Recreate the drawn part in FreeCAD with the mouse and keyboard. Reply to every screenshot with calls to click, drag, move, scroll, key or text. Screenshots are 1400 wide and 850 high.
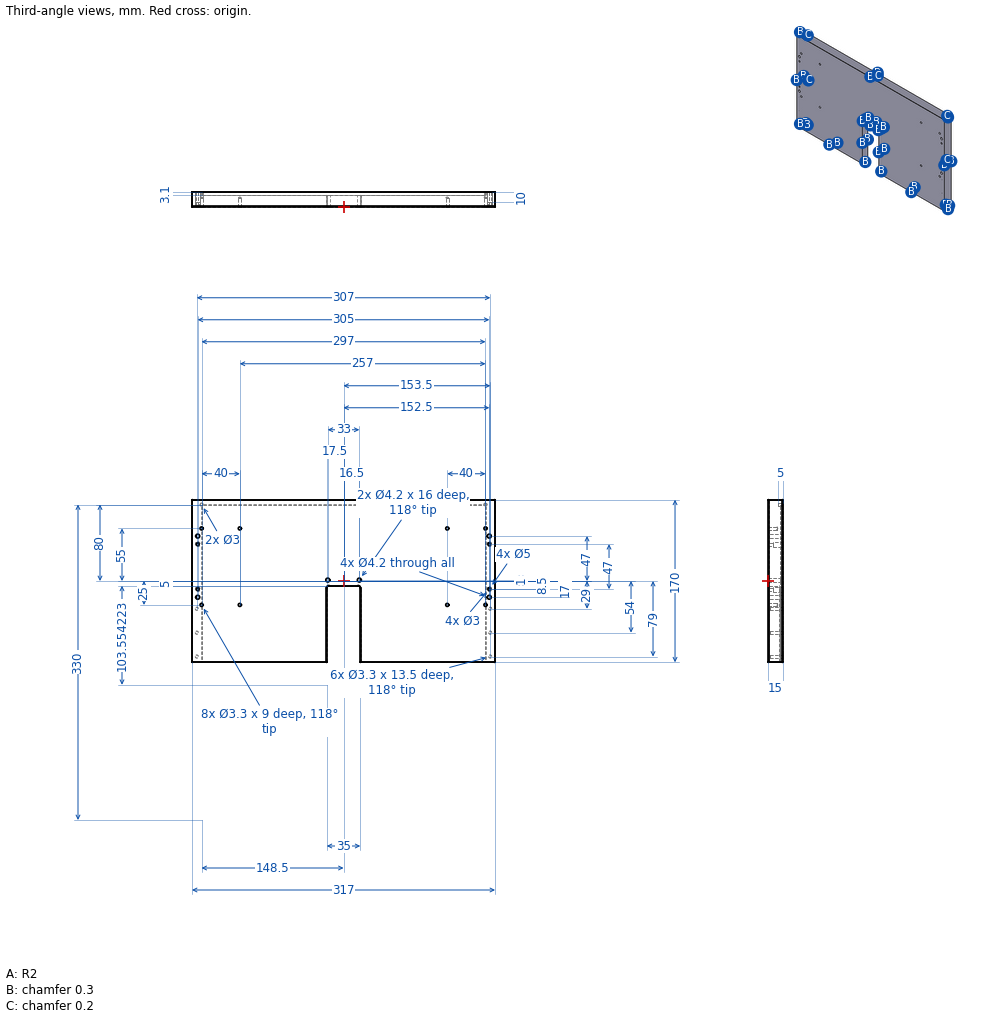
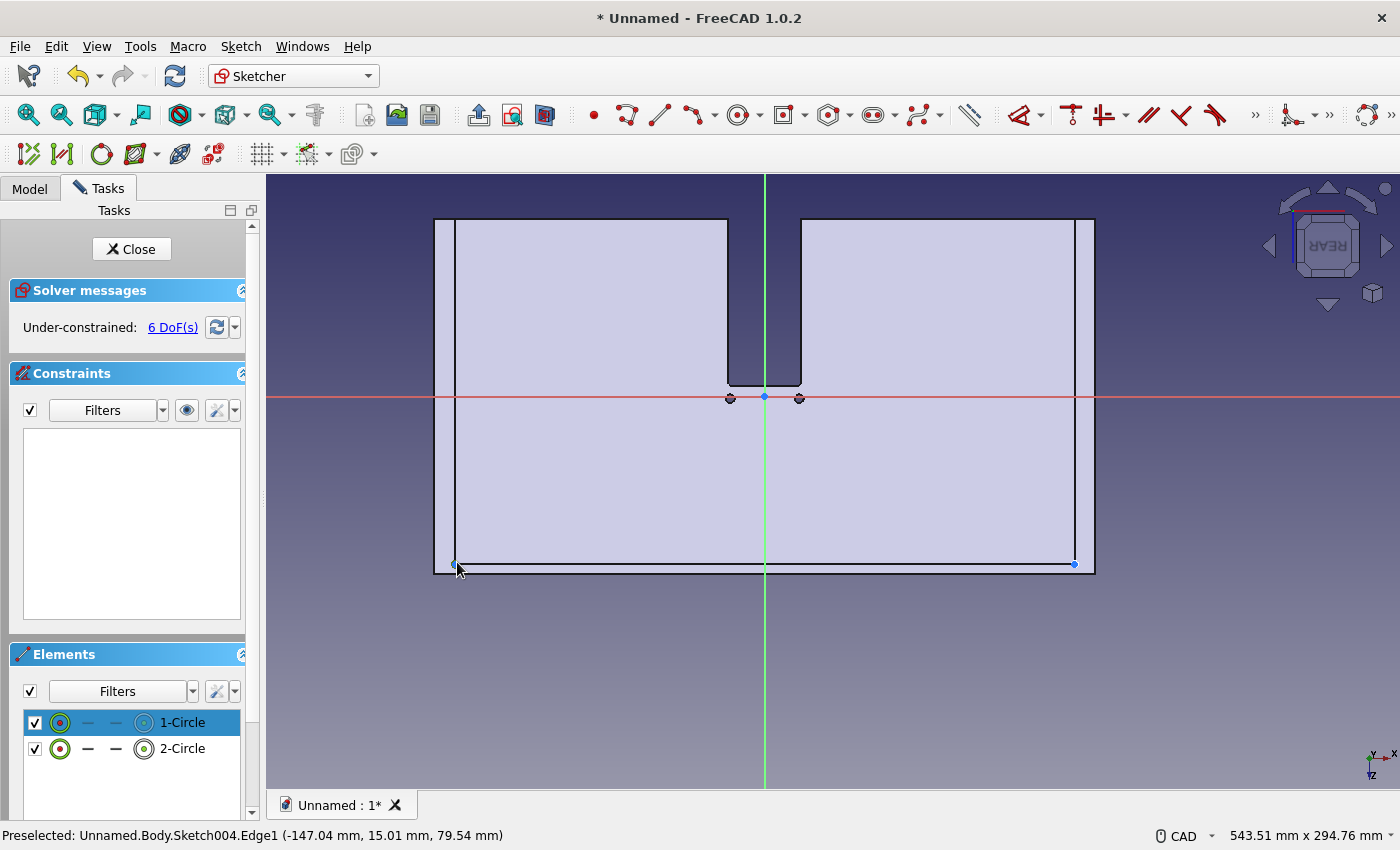
scroll(1077, 562, up, 8)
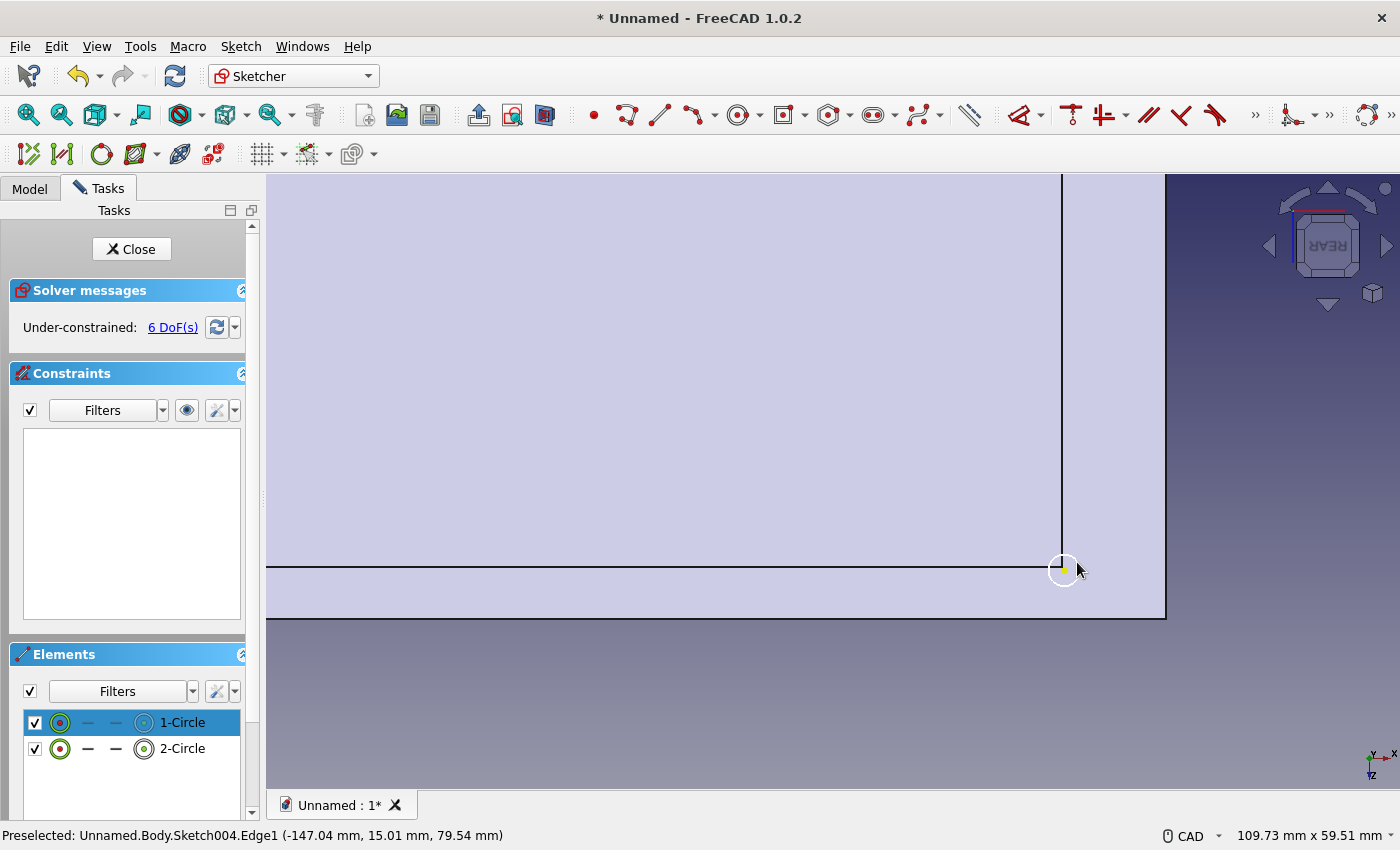
click(1075, 559)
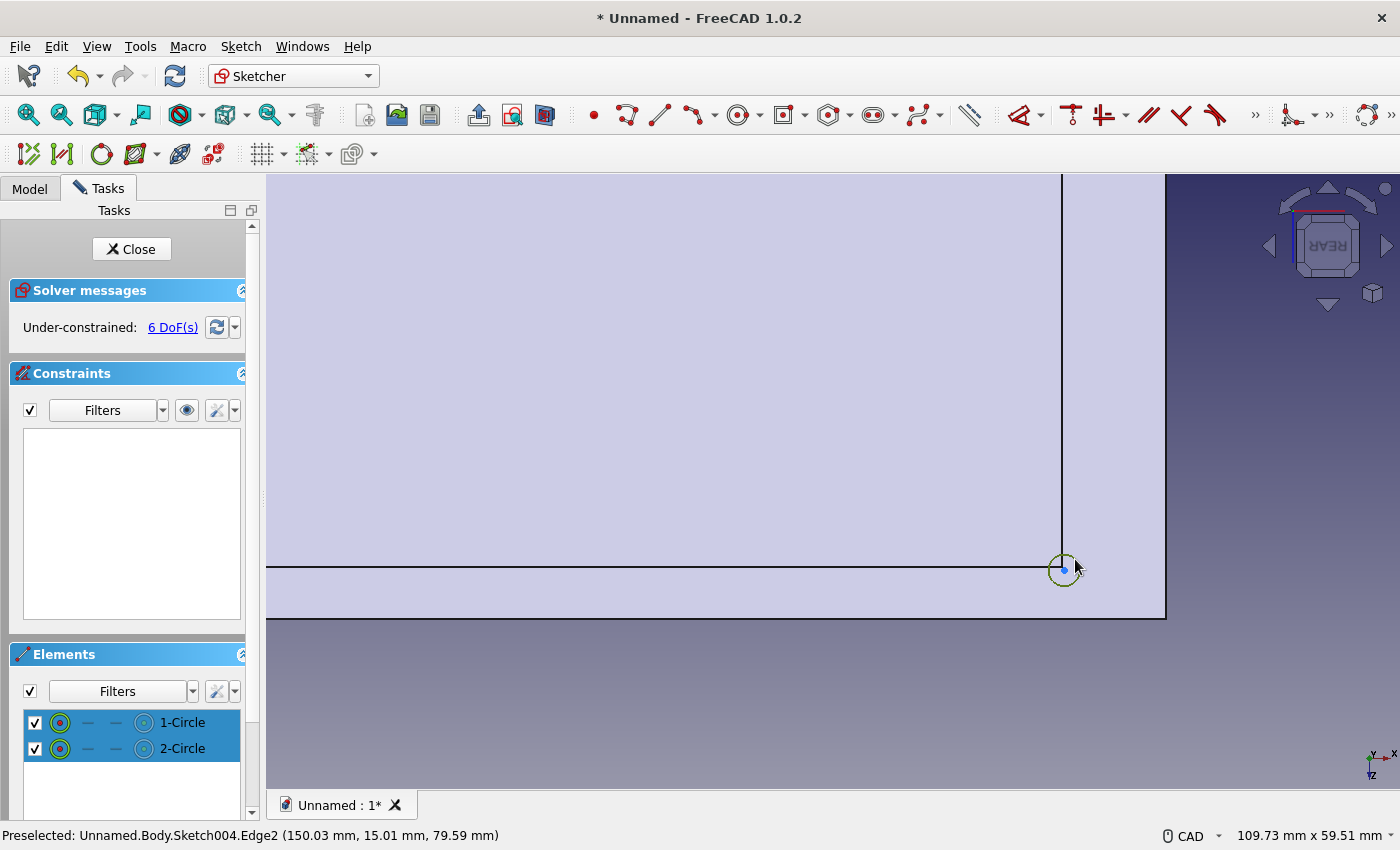
key(e)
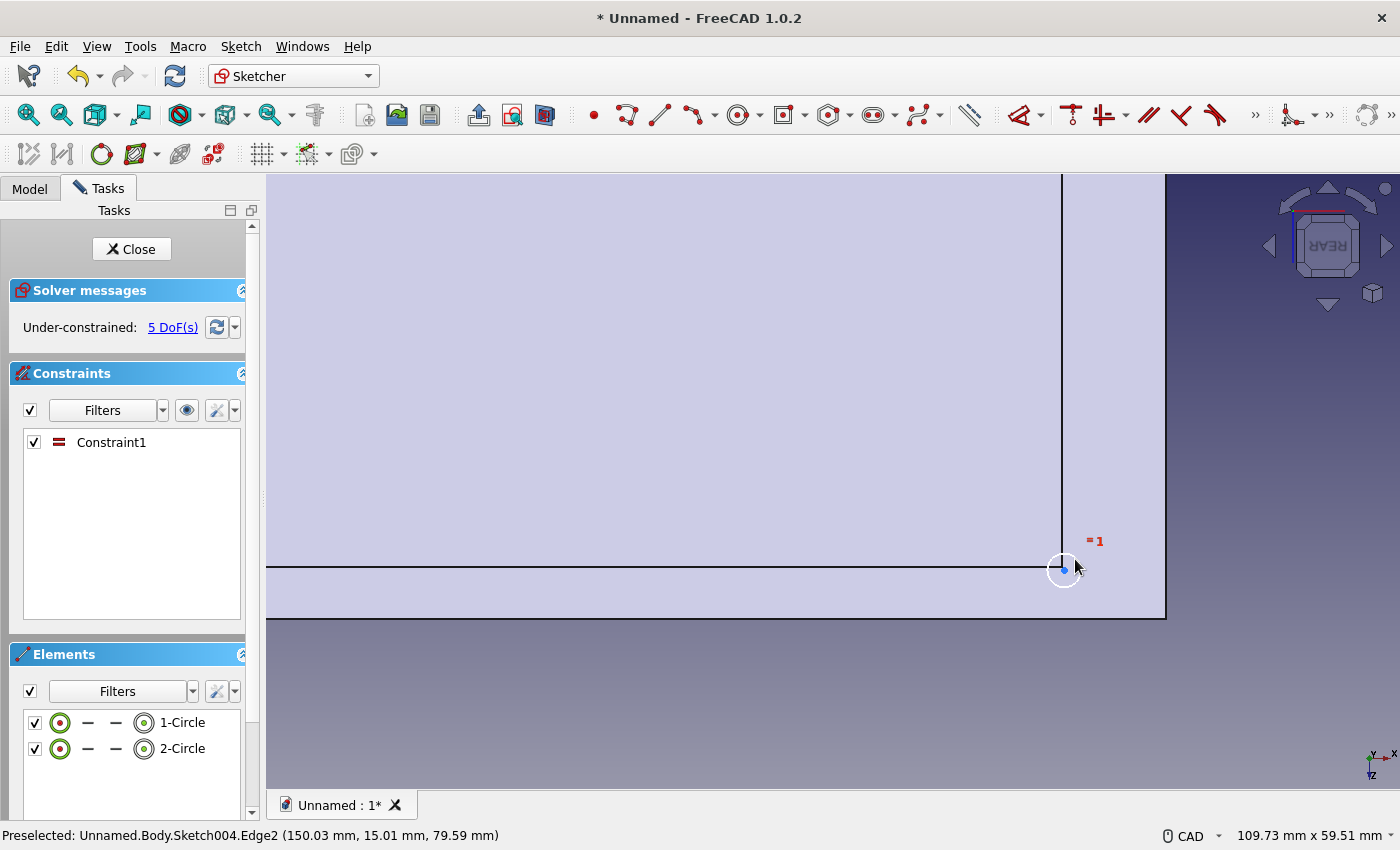
scroll(1077, 562, down, 8)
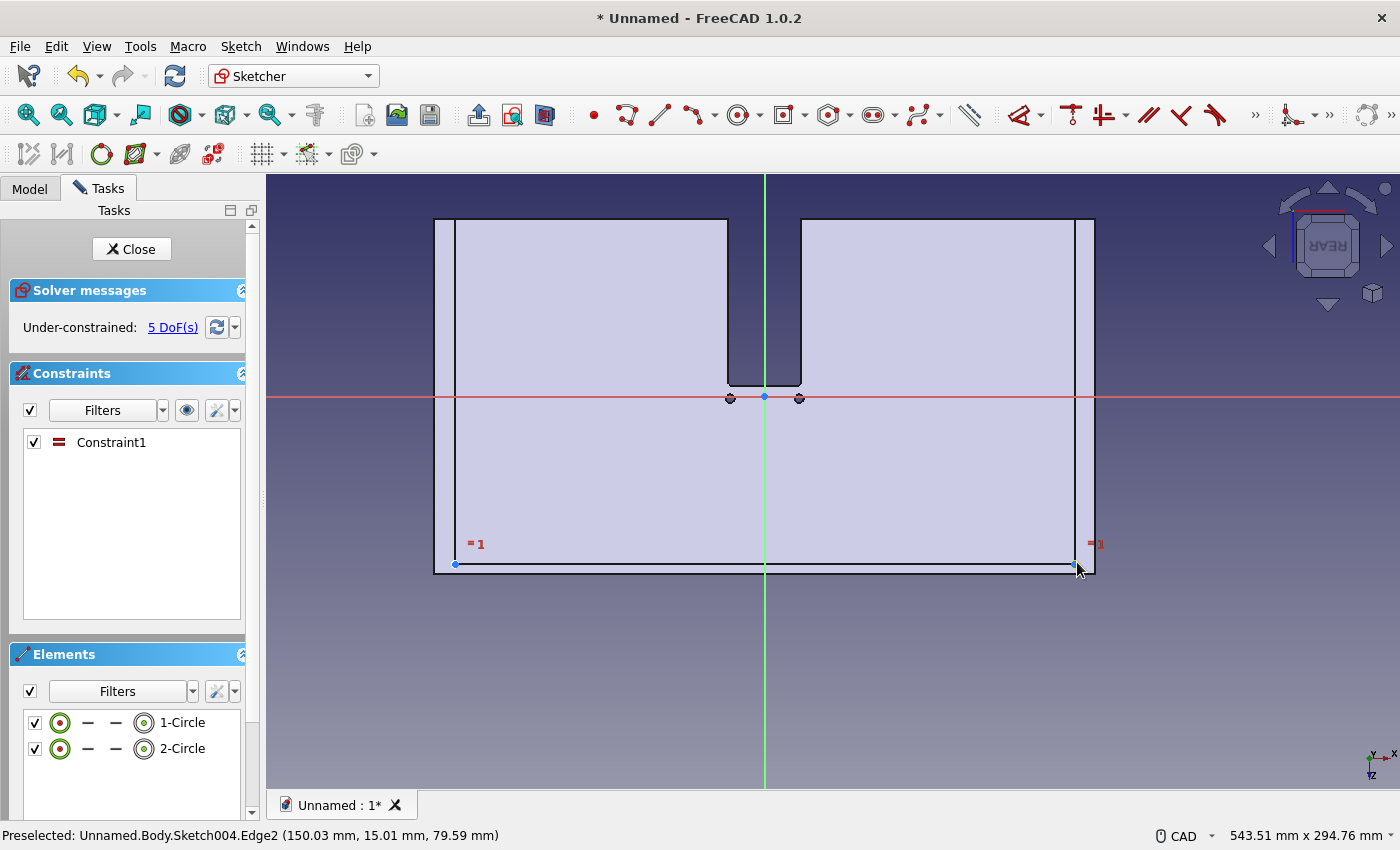
click(455, 564)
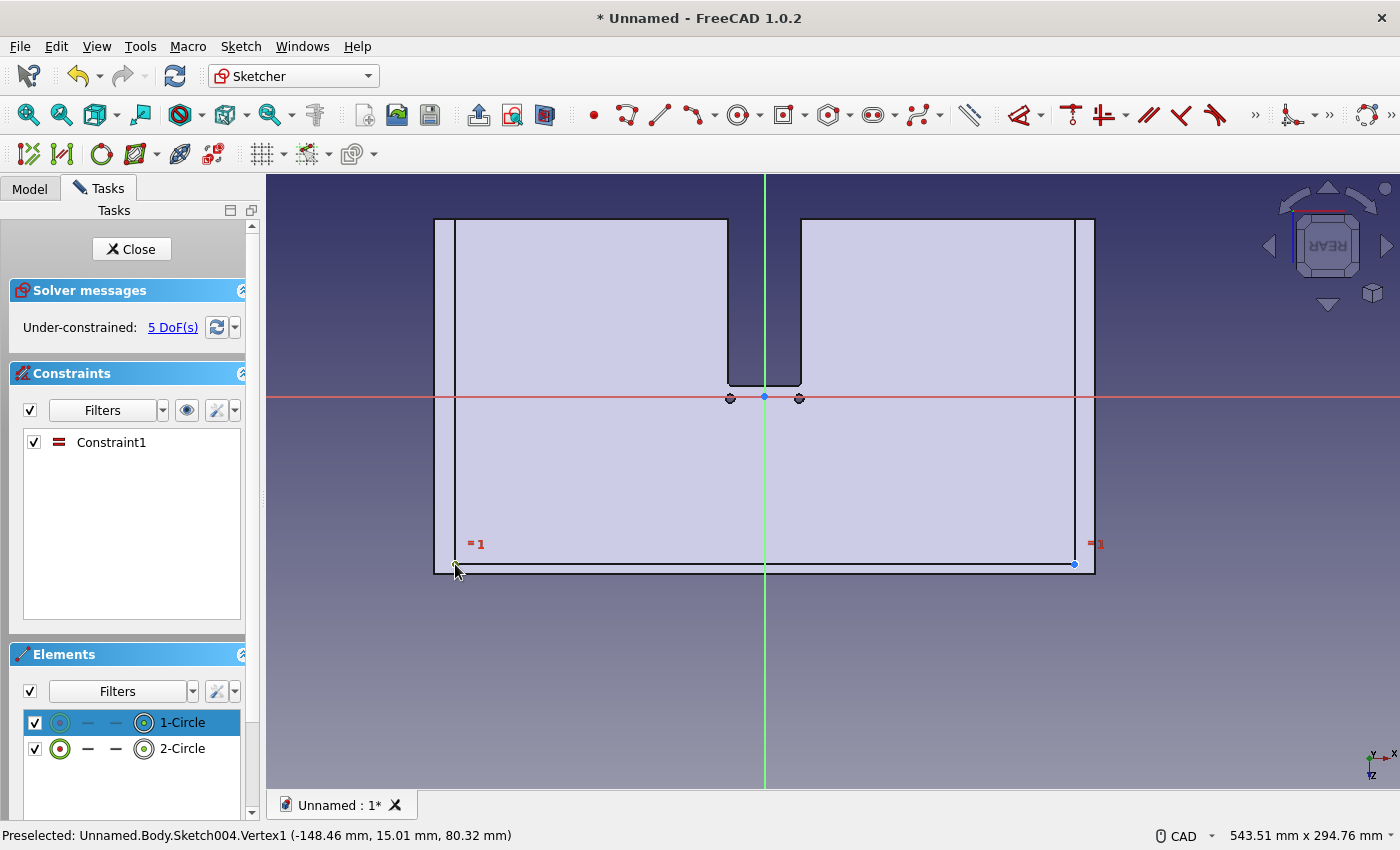
click(1075, 564)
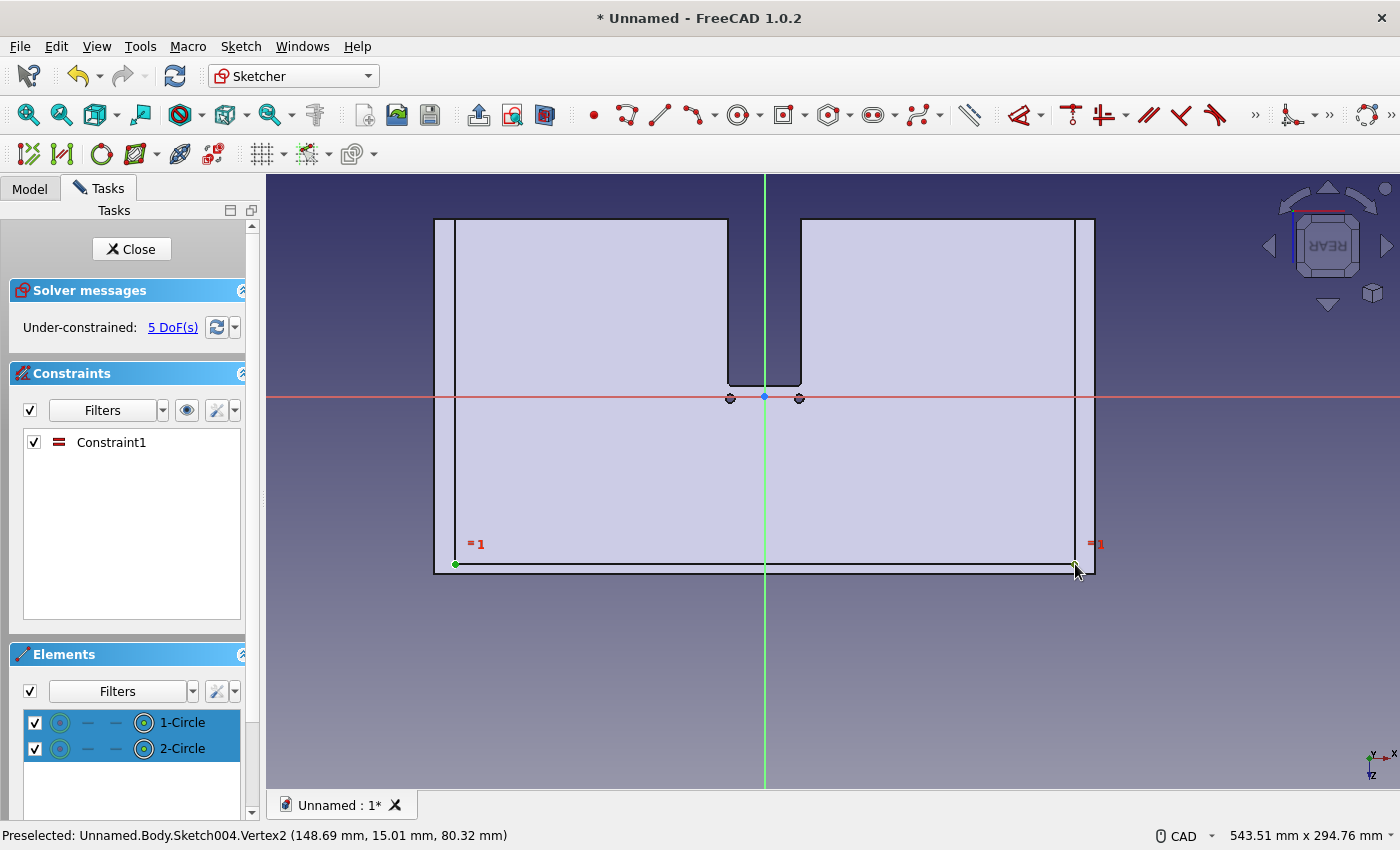
key(h)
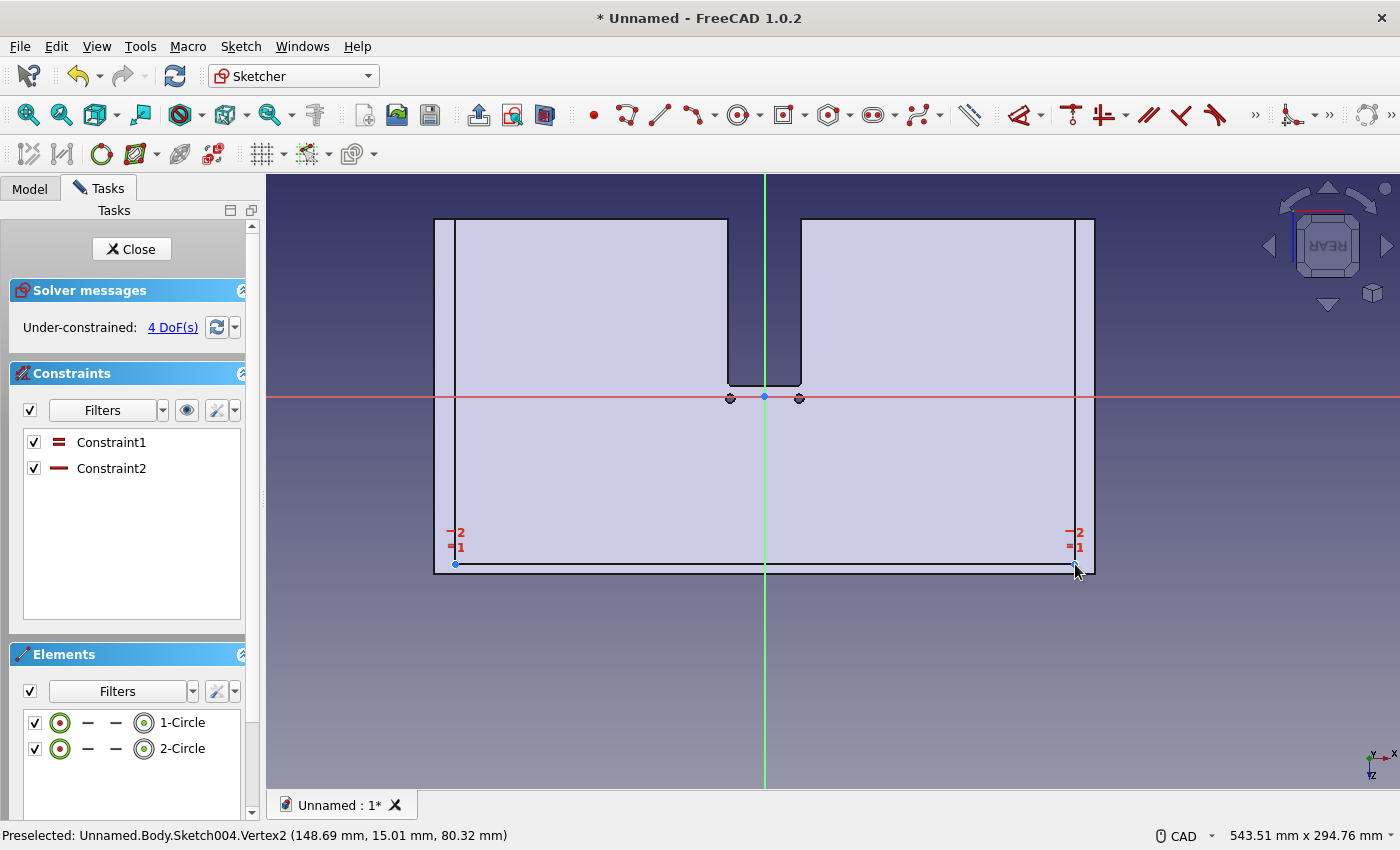
key(d)